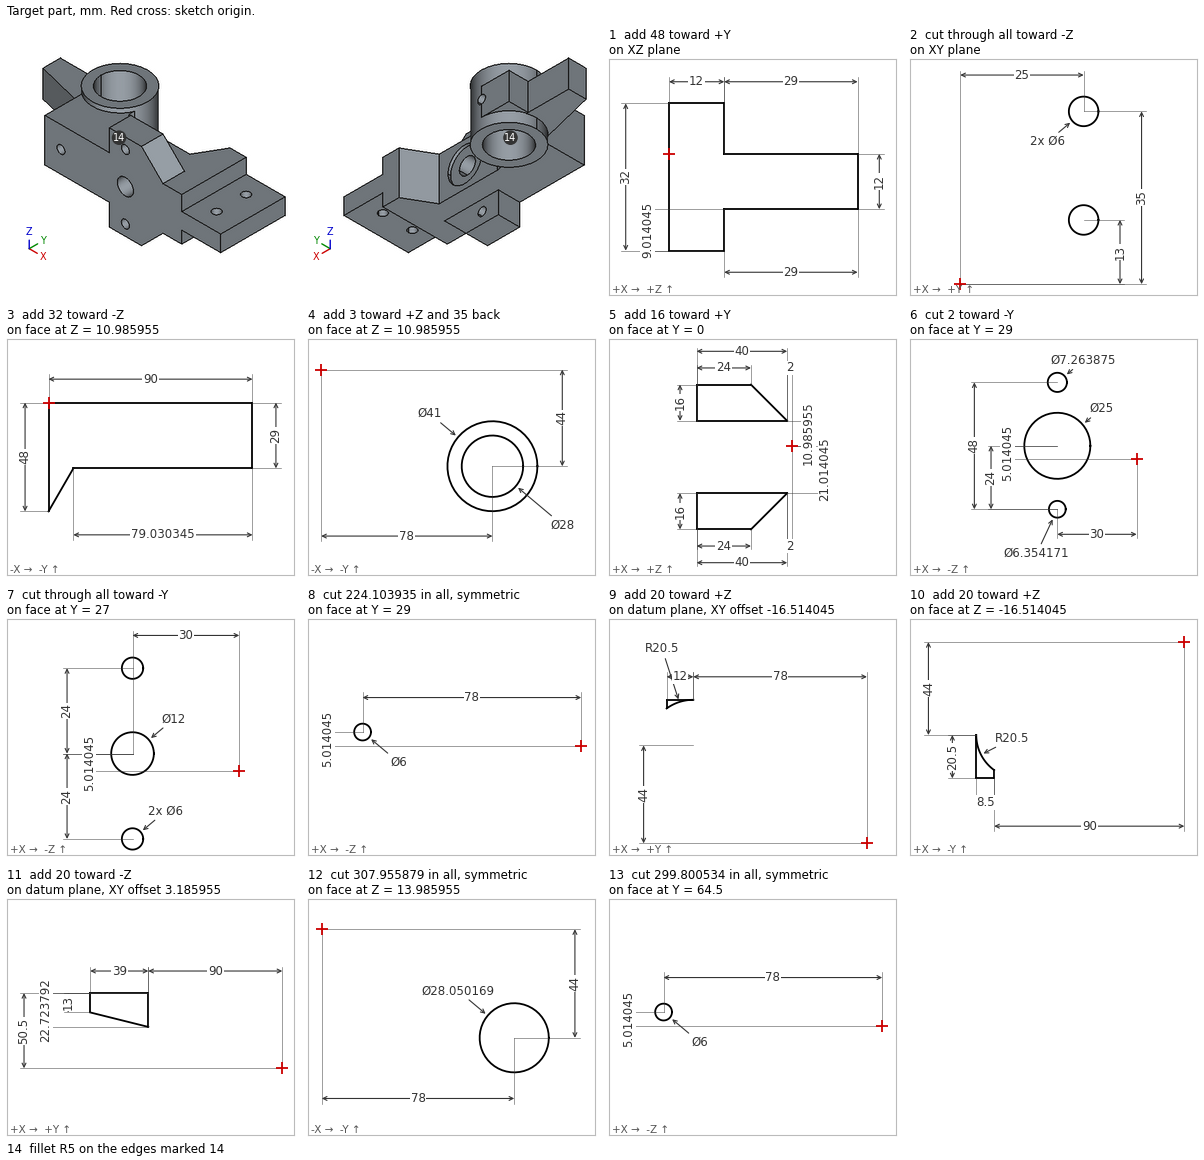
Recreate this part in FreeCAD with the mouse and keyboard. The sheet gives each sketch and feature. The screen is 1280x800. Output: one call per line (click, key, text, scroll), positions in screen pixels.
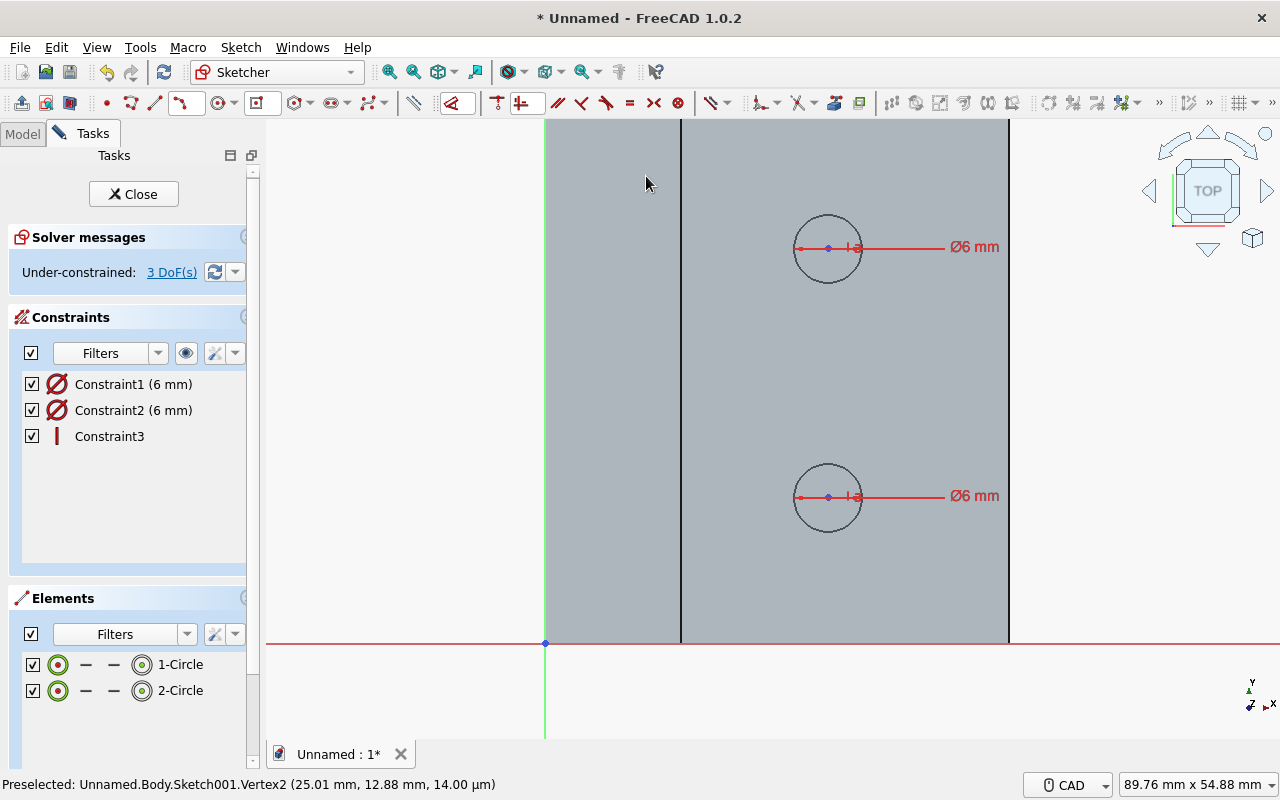
click(828, 249)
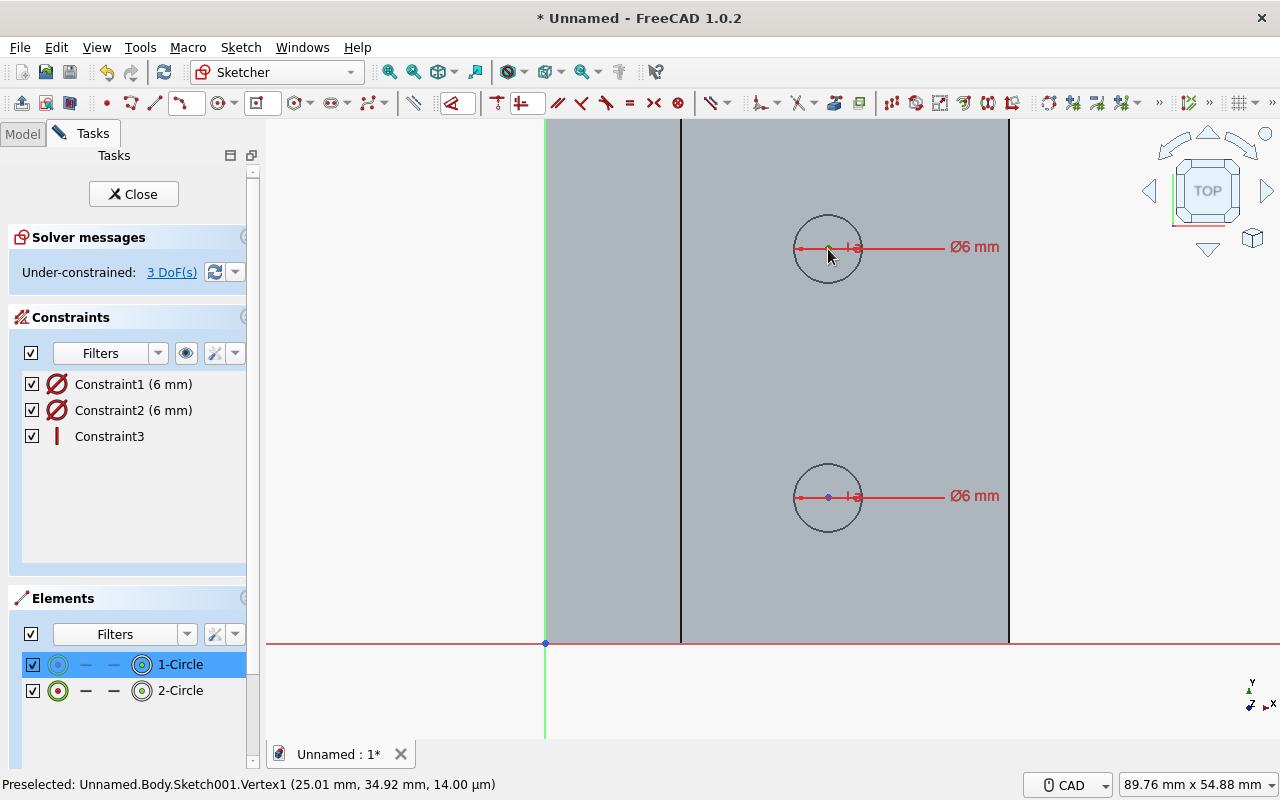
key(l)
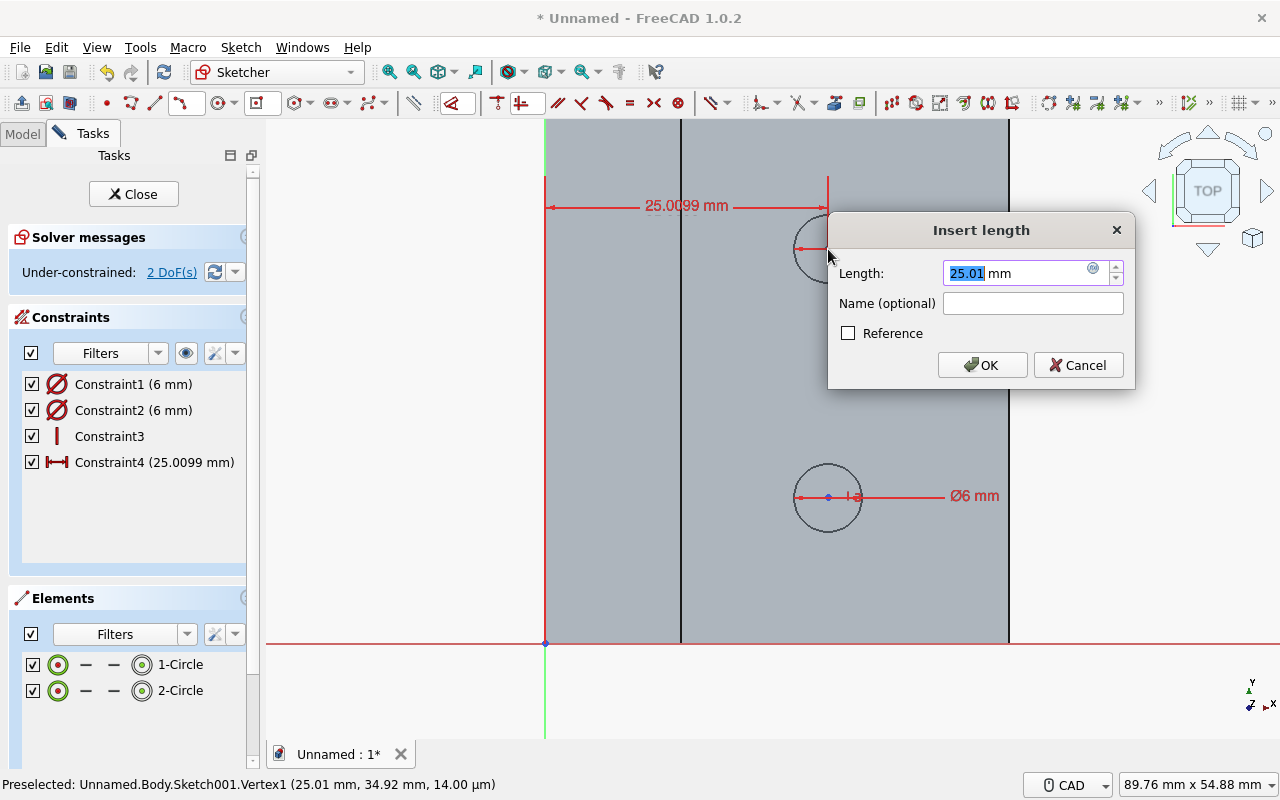
text(25)
key(Return)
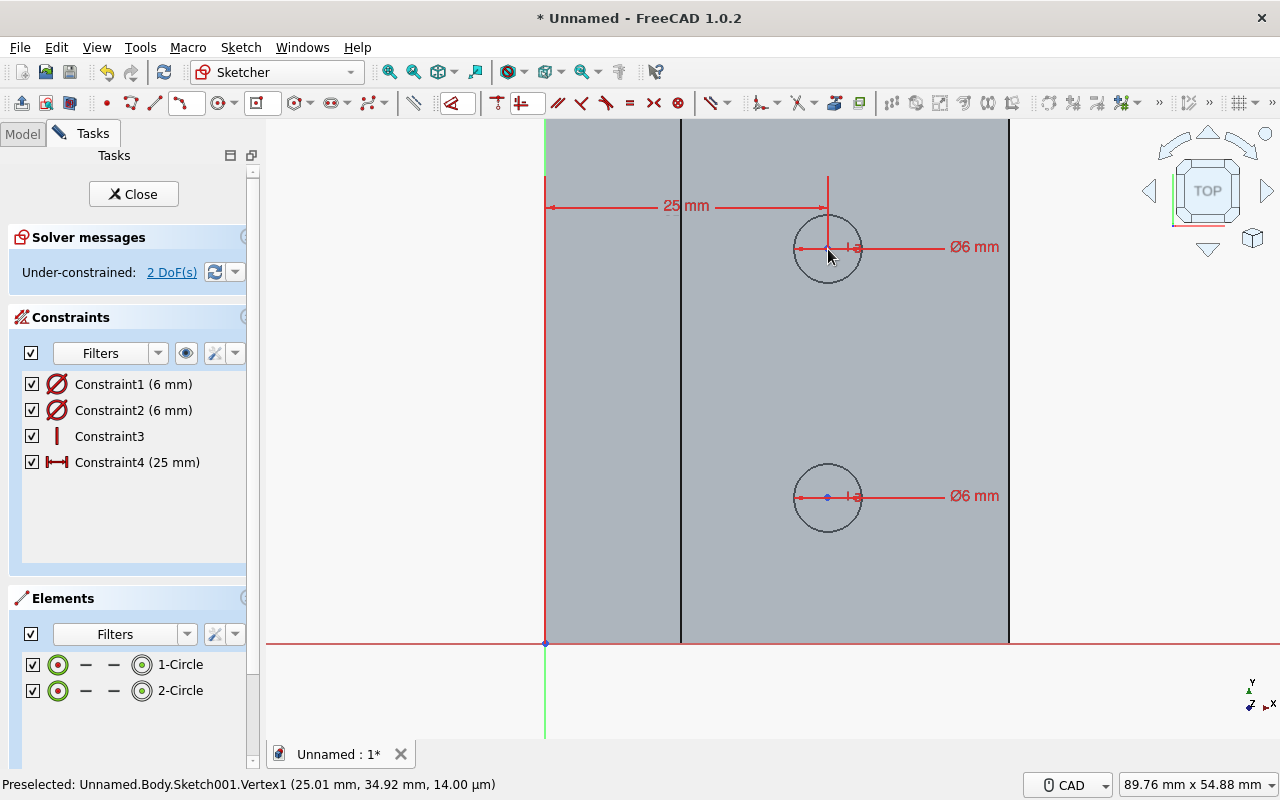
click(828, 249)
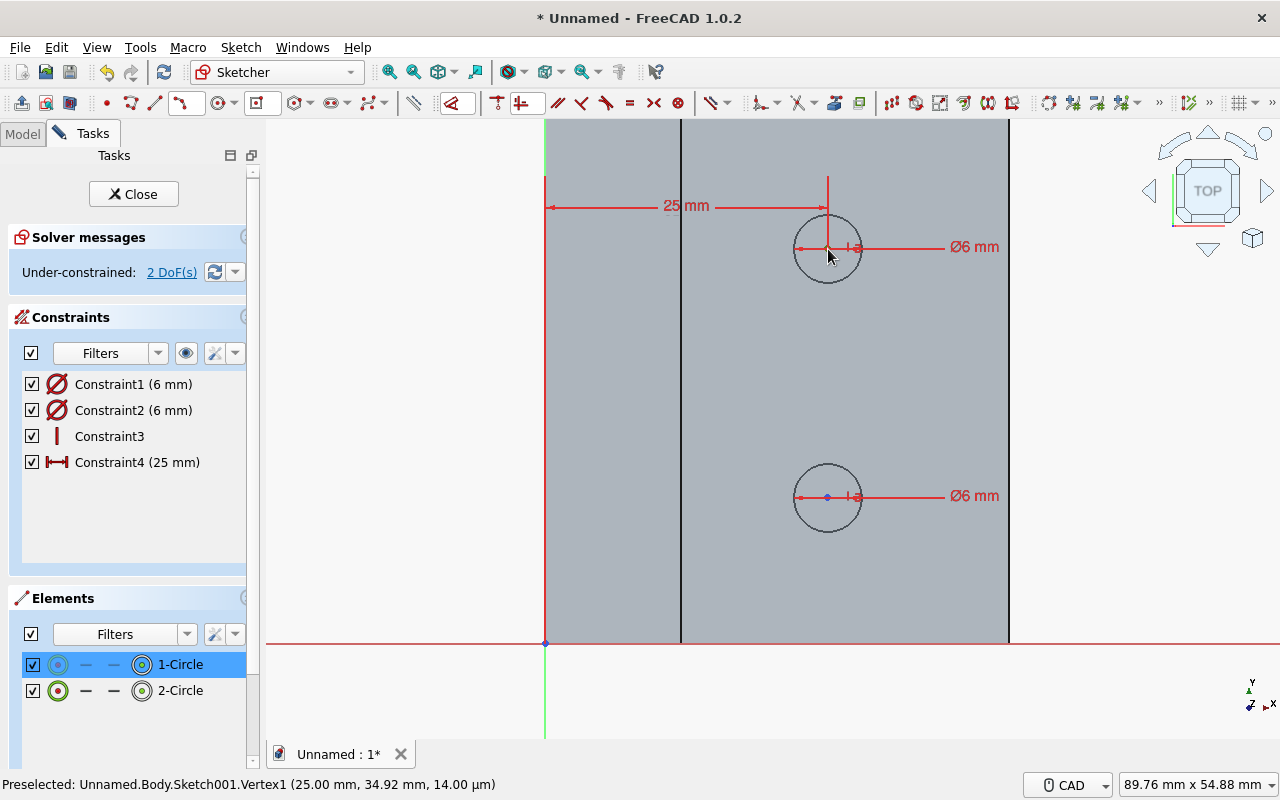
key(i)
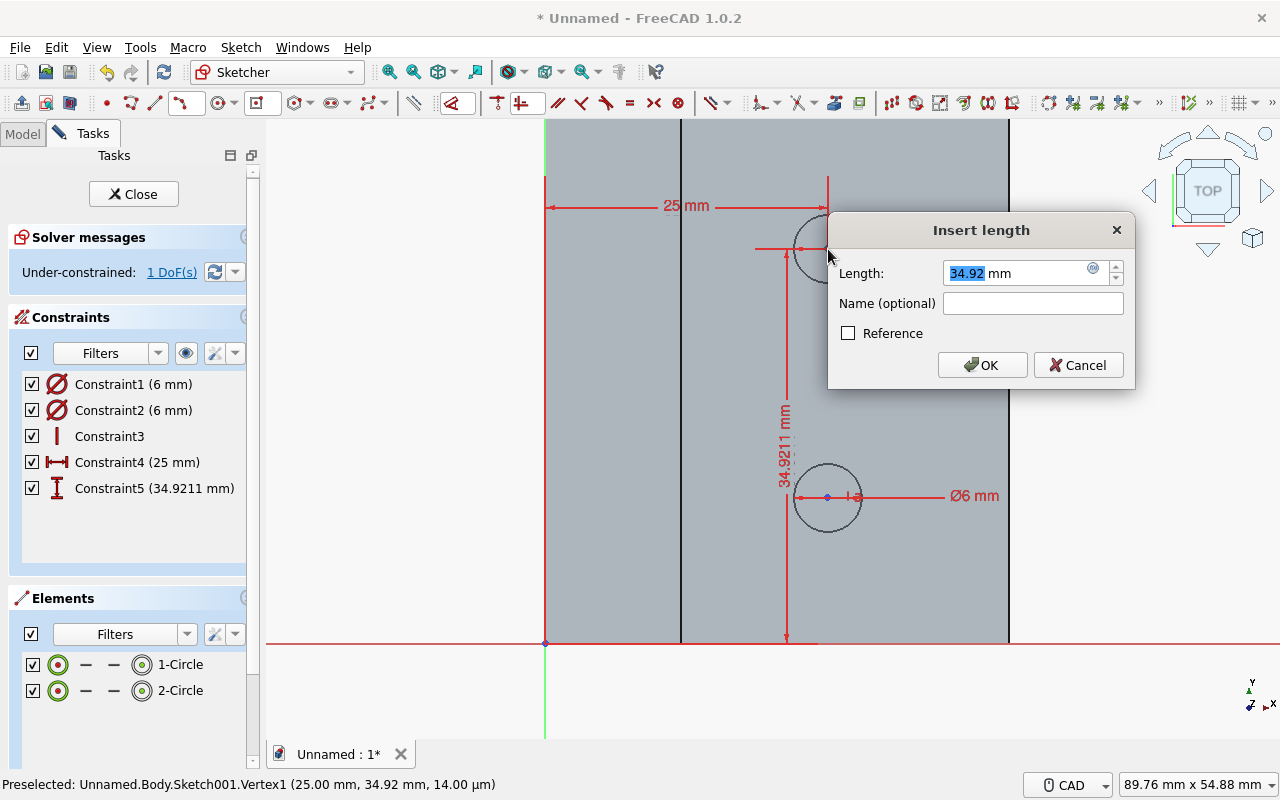
text(35)
key(Return)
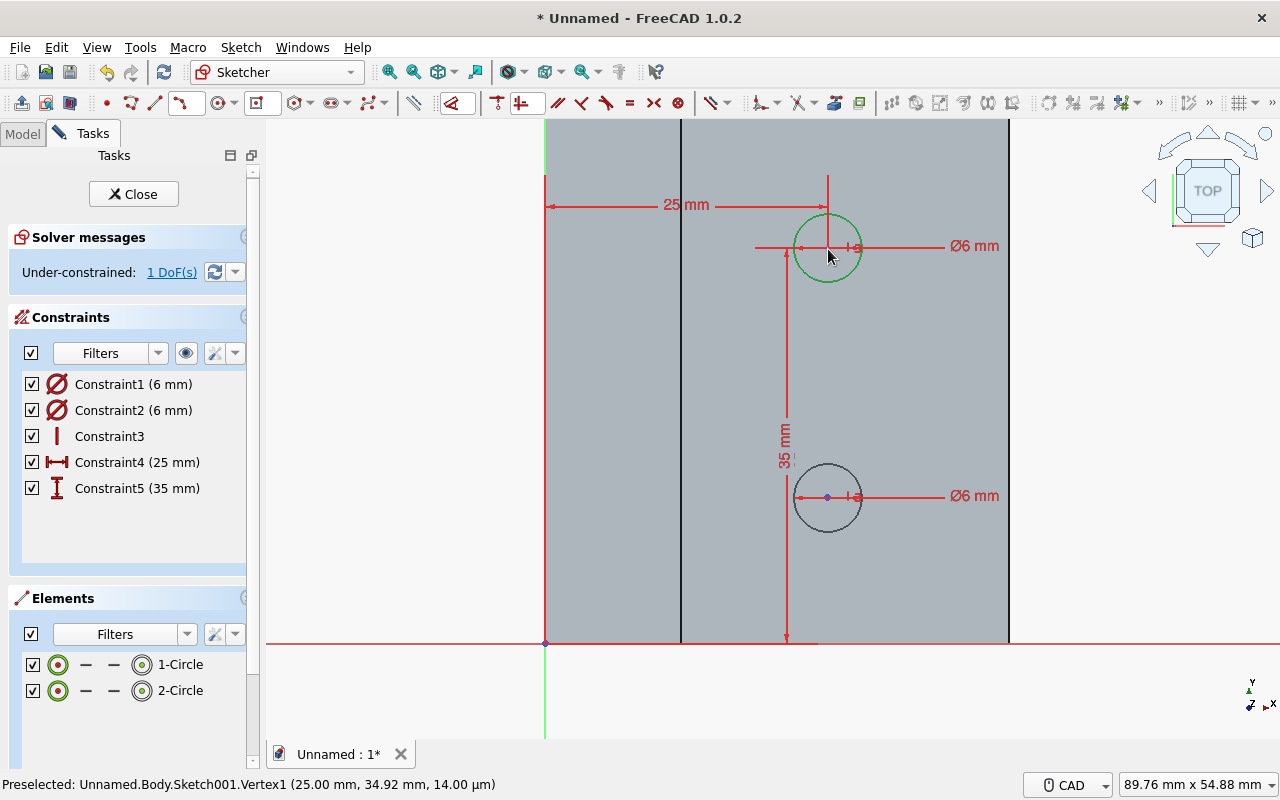
click(828, 498)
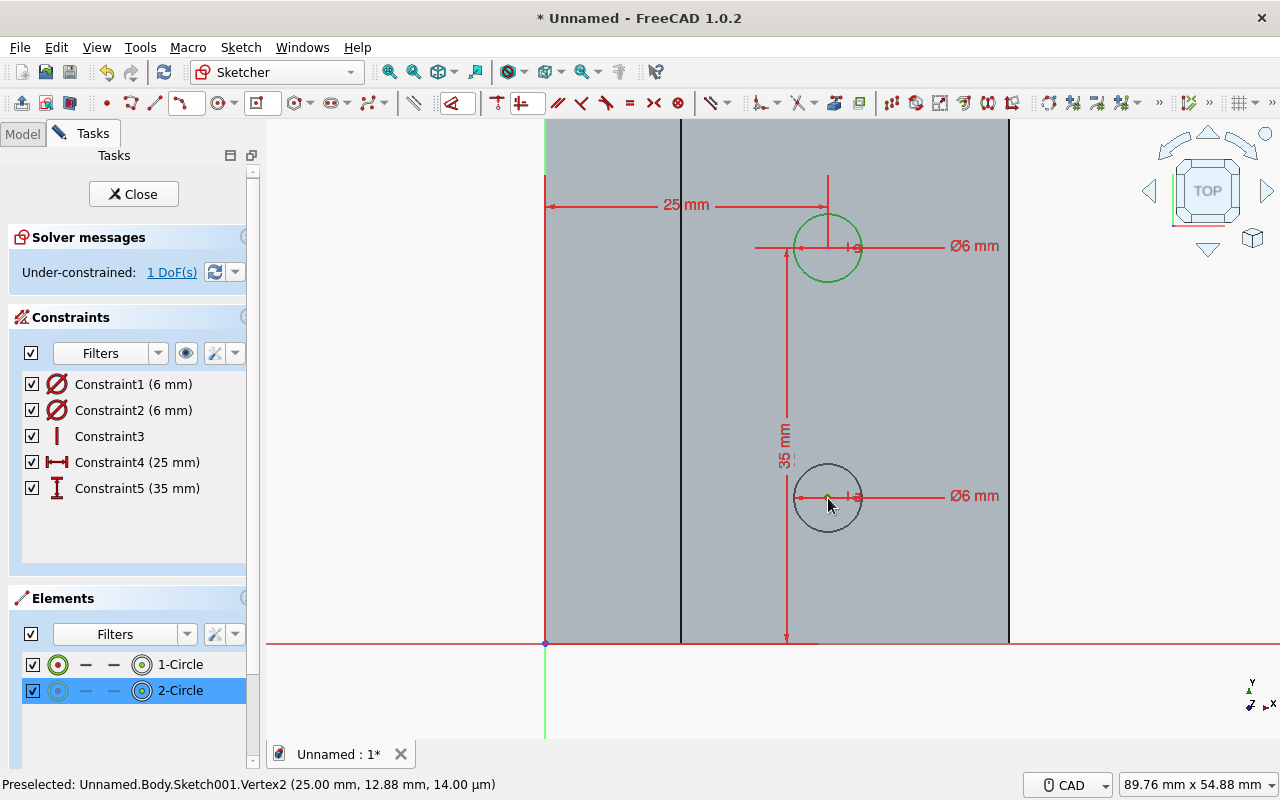
key(i)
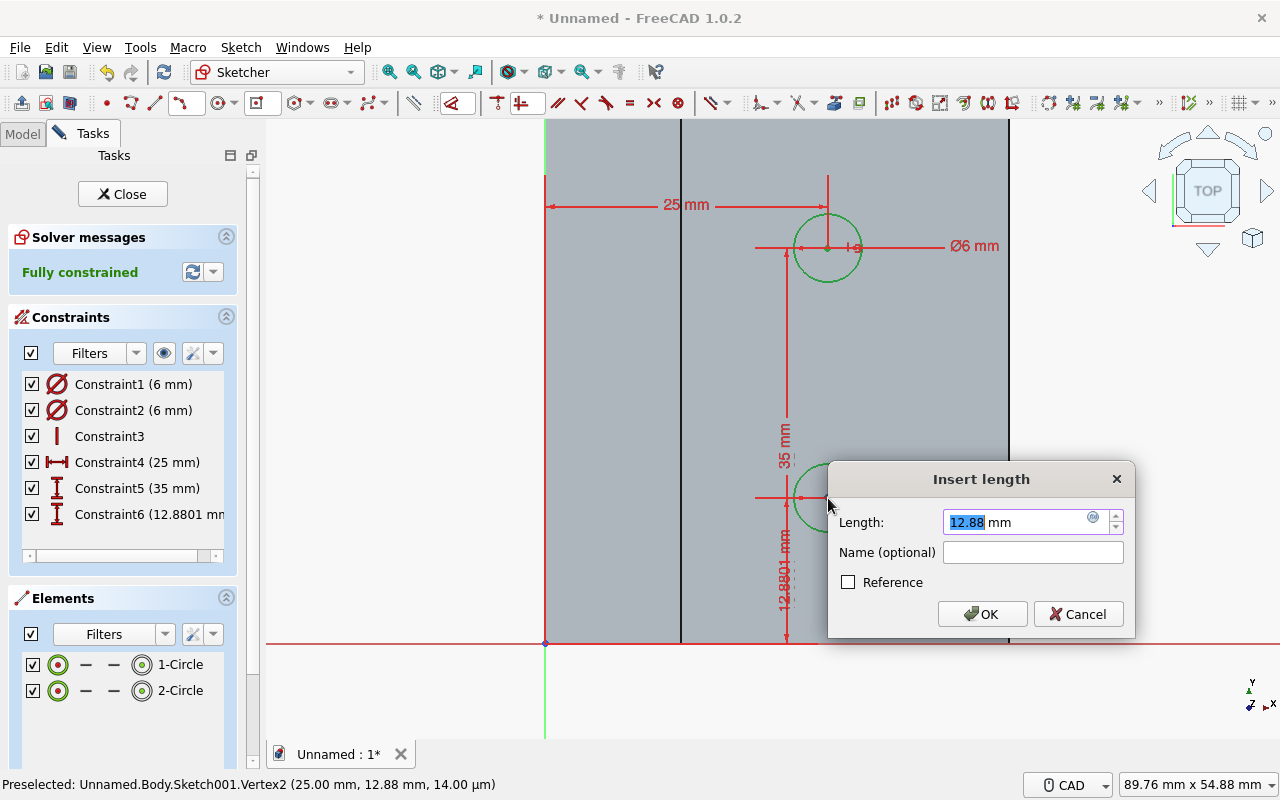
text(13)
key(Return)